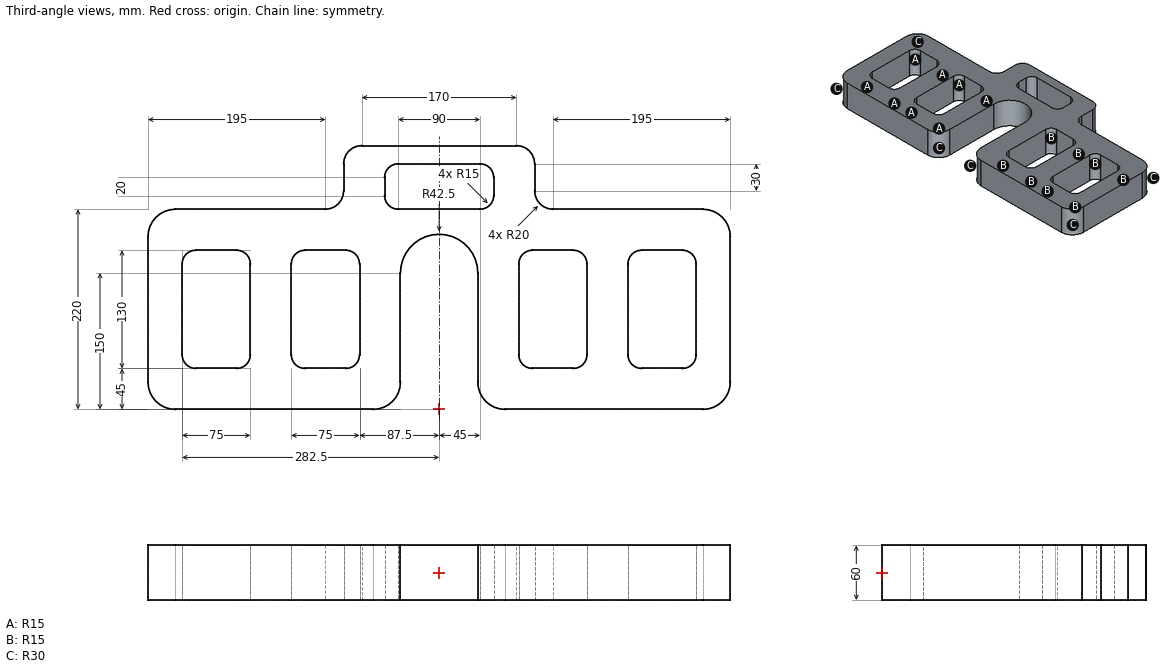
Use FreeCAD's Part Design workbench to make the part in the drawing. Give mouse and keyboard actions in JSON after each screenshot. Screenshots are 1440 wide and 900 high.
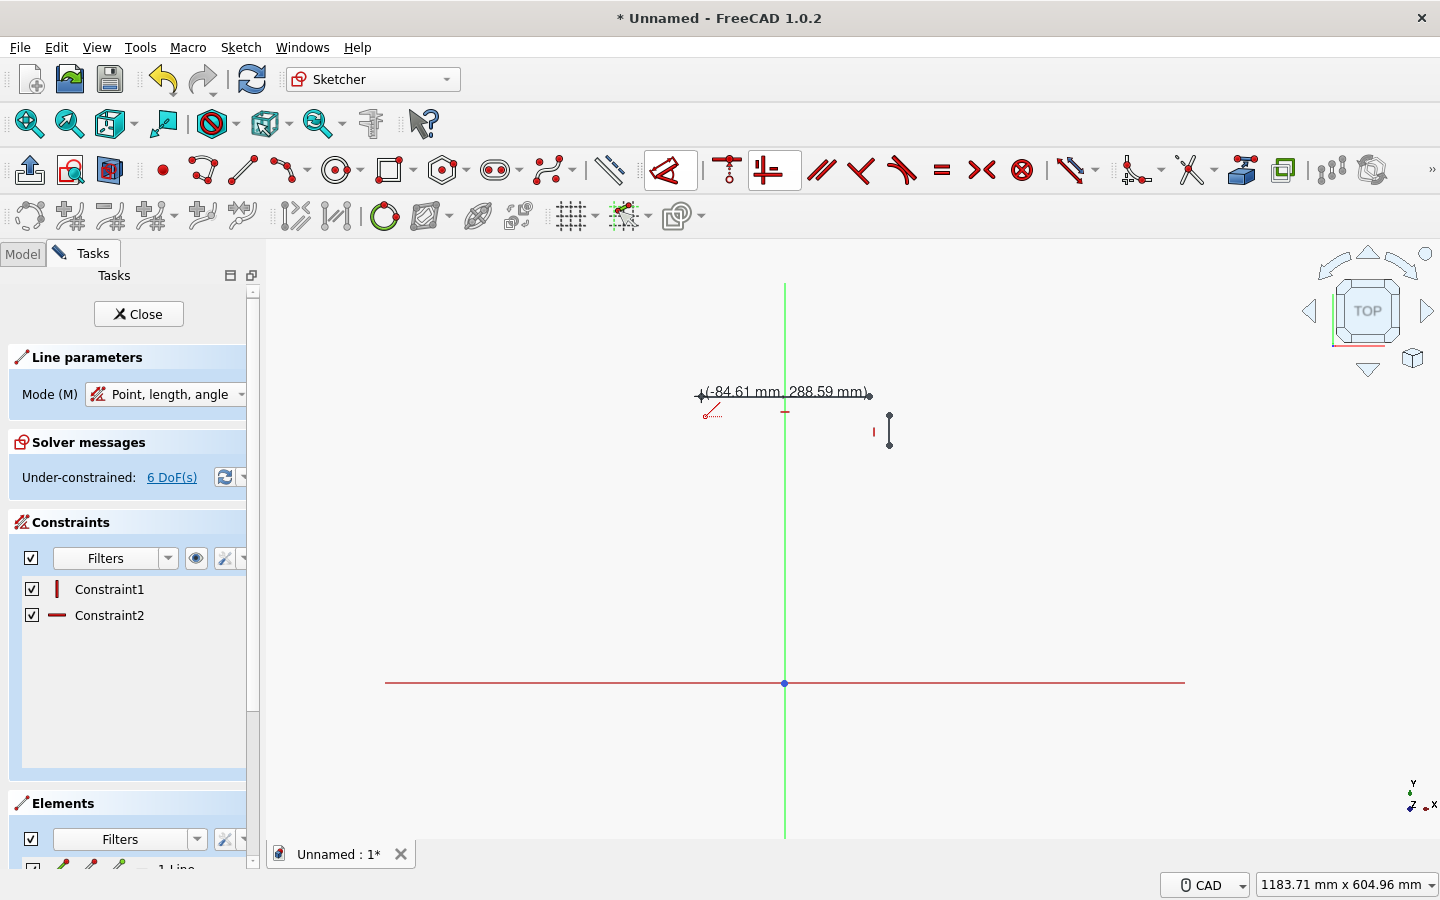
{"action": "left_click", "coordinate": [681, 415]}
{"action": "left_click", "coordinate": [681, 445]}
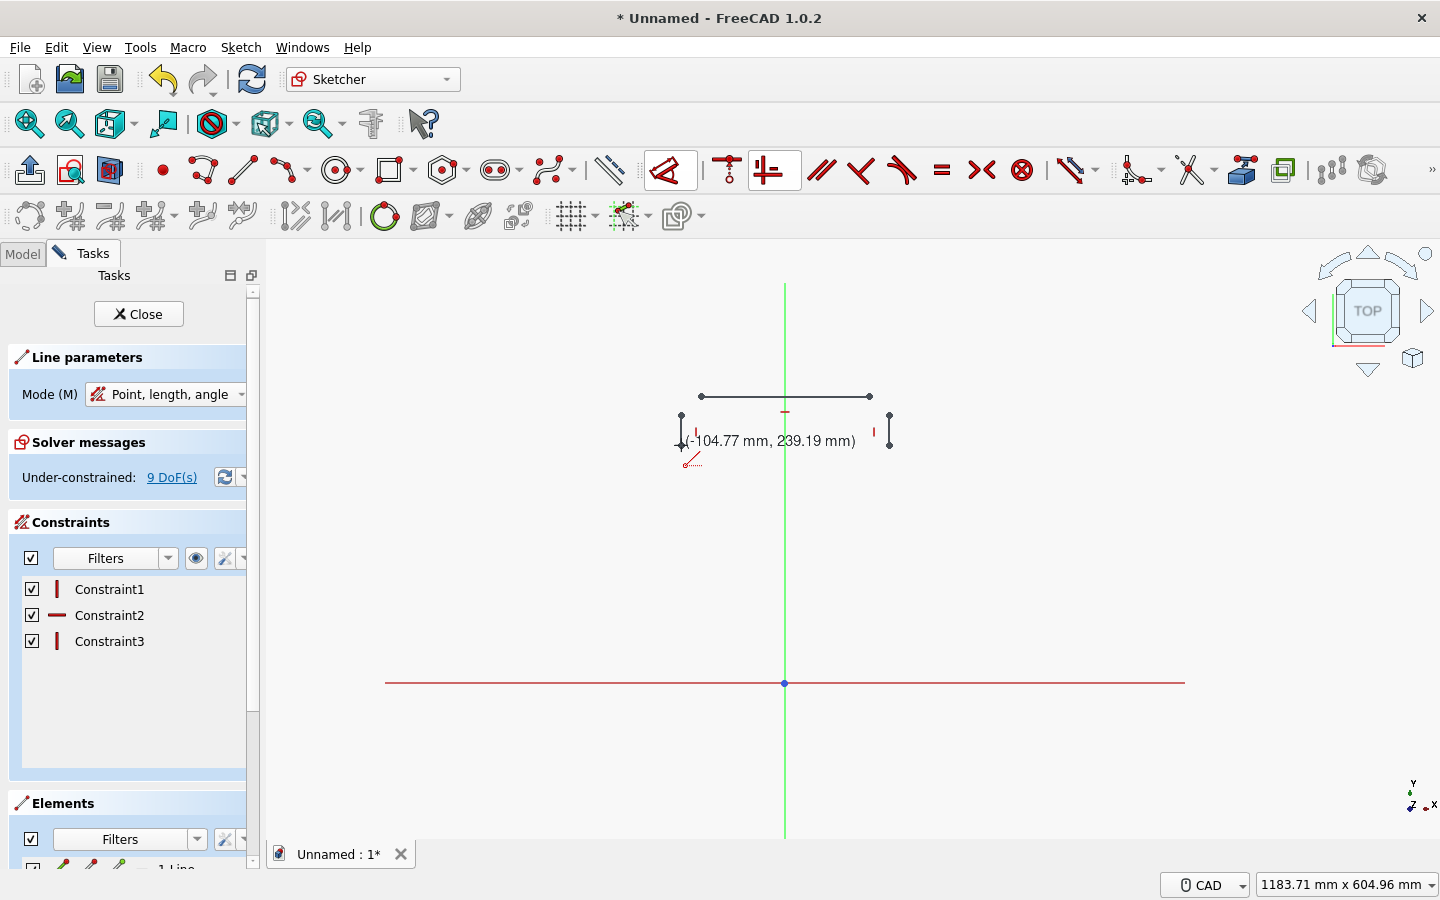
{"action": "left_click", "coordinate": [204, 170]}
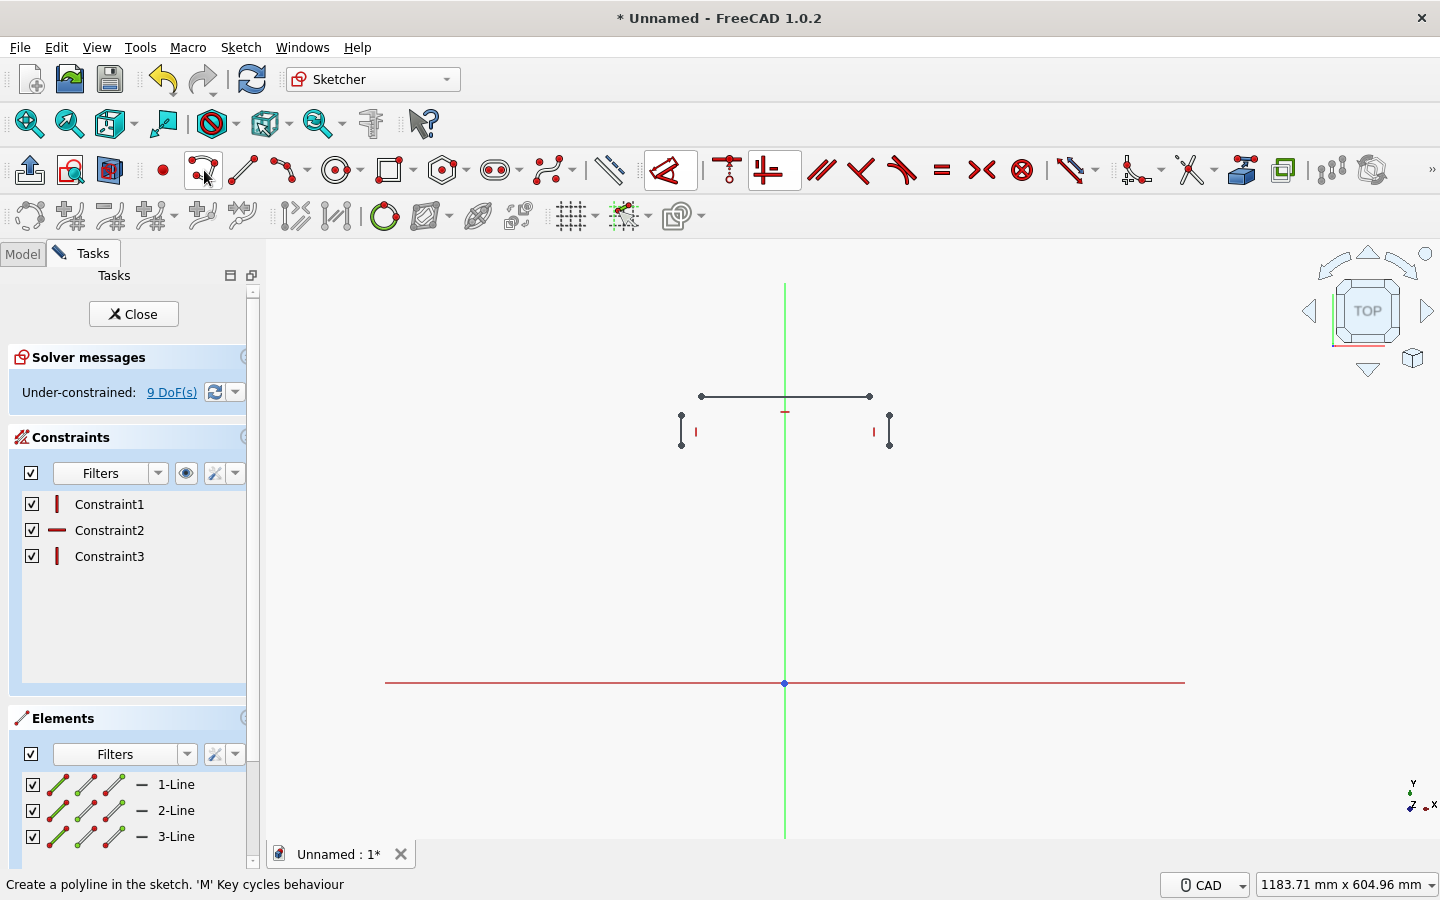
{"action": "left_click", "coordinate": [661, 465]}
{"action": "left_click", "coordinate": [468, 465]}
{"action": "left_click", "coordinate": [468, 683]}
{"action": "left_click", "coordinate": [743, 674]}
{"action": "left_click", "coordinate": [743, 534]}
{"action": "right_click", "coordinate": [743, 534]}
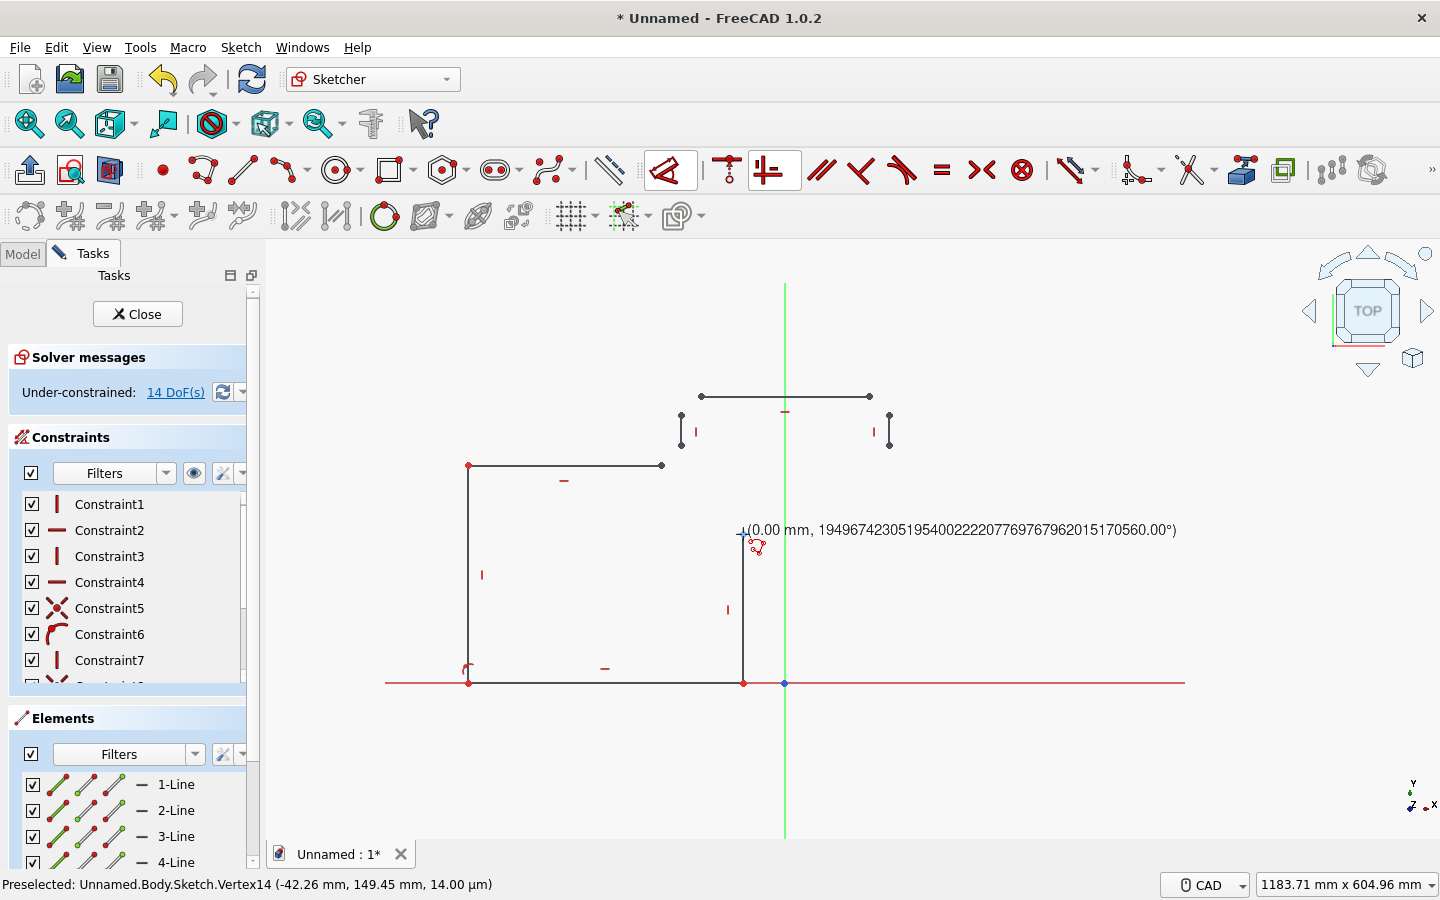
{"action": "left_click", "coordinate": [827, 534]}
{"action": "left_click", "coordinate": [827, 683]}
{"action": "left_click", "coordinate": [1102, 674]}
{"action": "left_click", "coordinate": [1102, 465]}
{"action": "left_click", "coordinate": [909, 465]}
{"action": "right_click", "coordinate": [909, 465]}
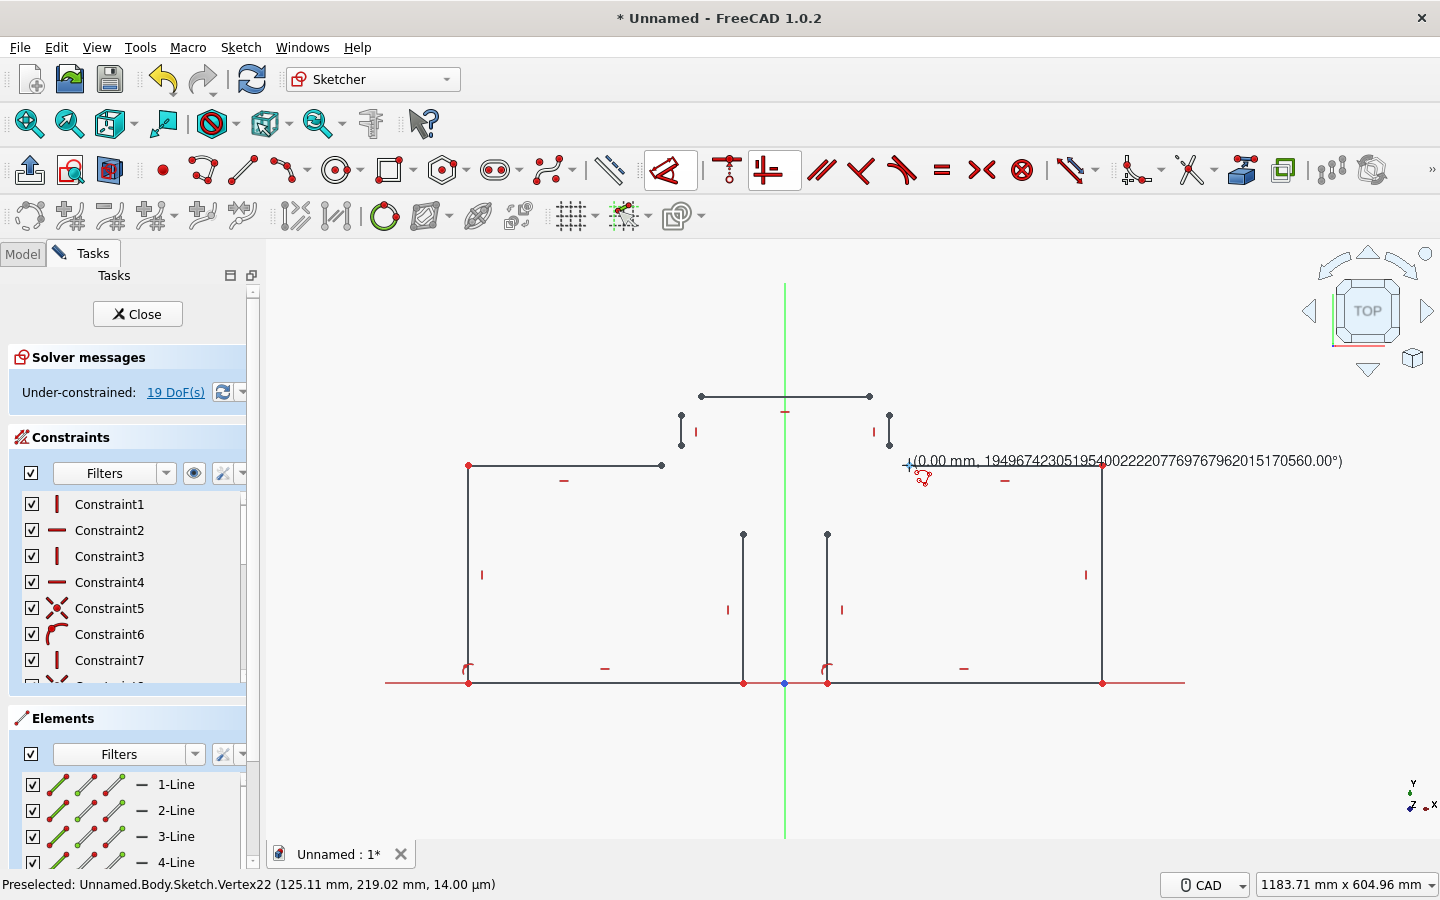
{"action": "left_click", "coordinate": [284, 170]}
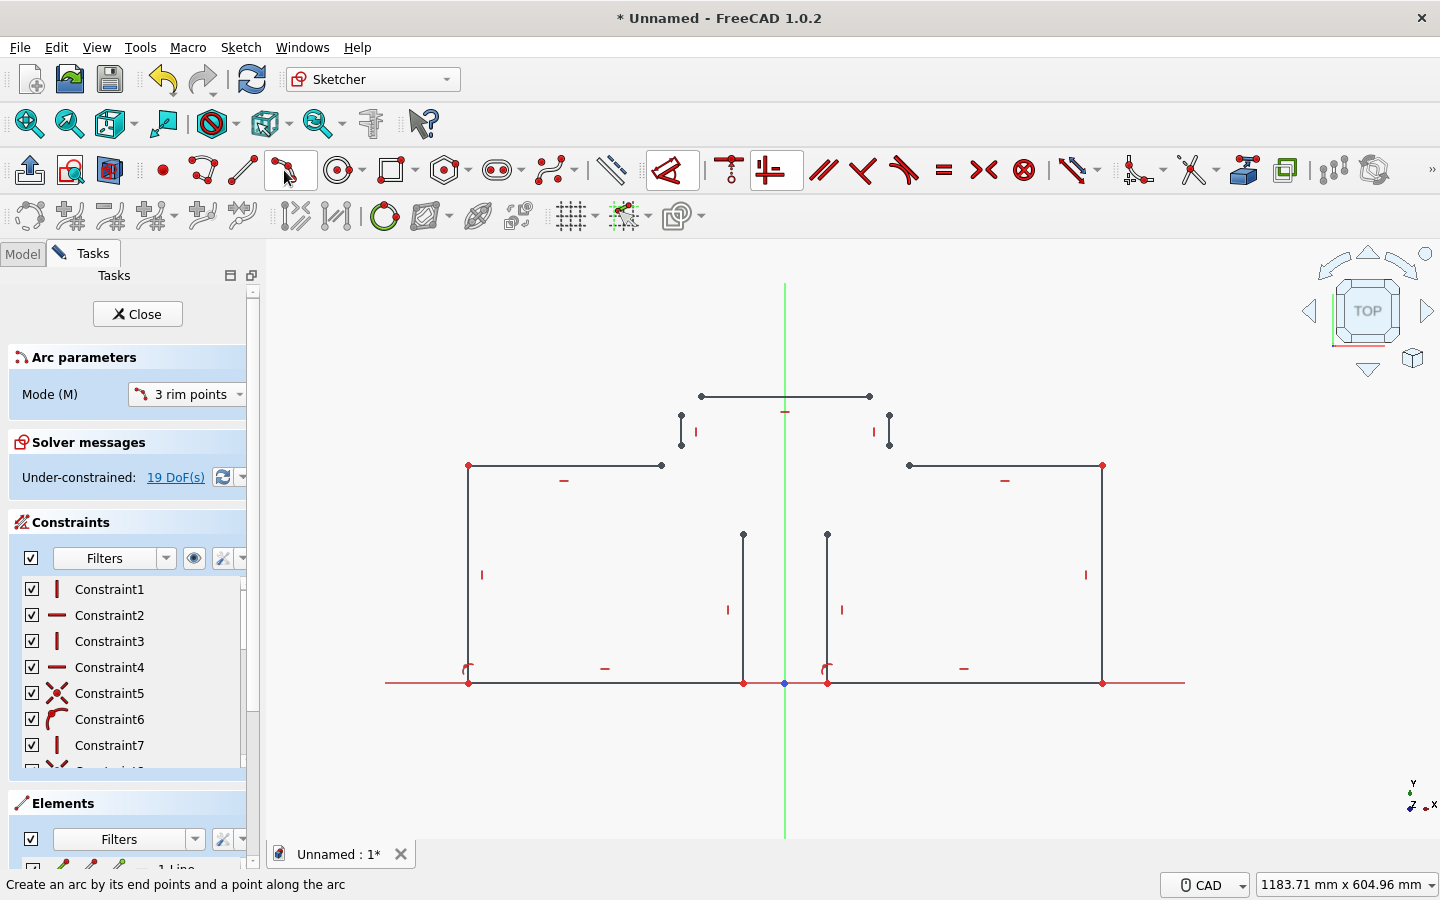
{"action": "left_click", "coordinate": [889, 416]}
{"action": "left_click", "coordinate": [869, 397]}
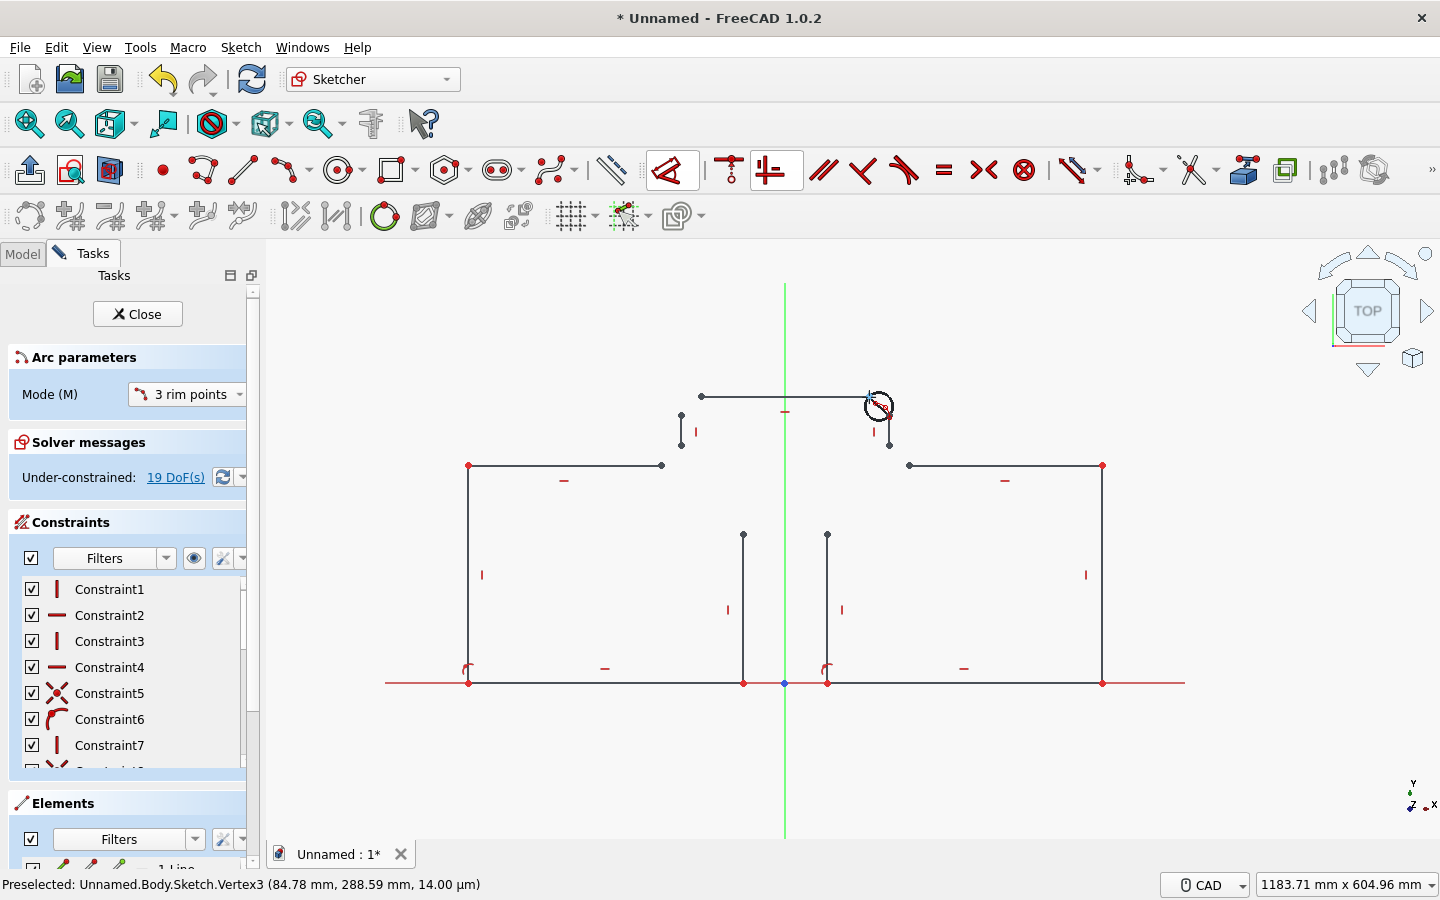
{"action": "scroll", "coordinate": [883, 401], "scroll_direction": "up", "scroll_amount": 6}